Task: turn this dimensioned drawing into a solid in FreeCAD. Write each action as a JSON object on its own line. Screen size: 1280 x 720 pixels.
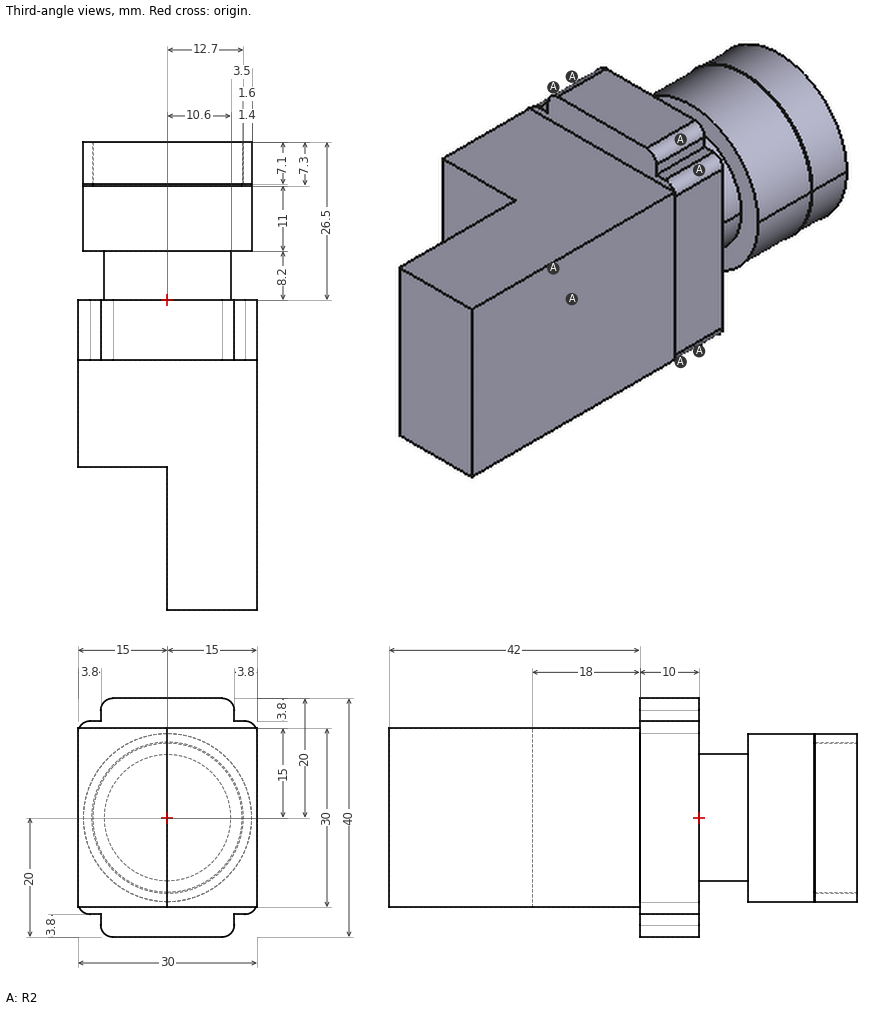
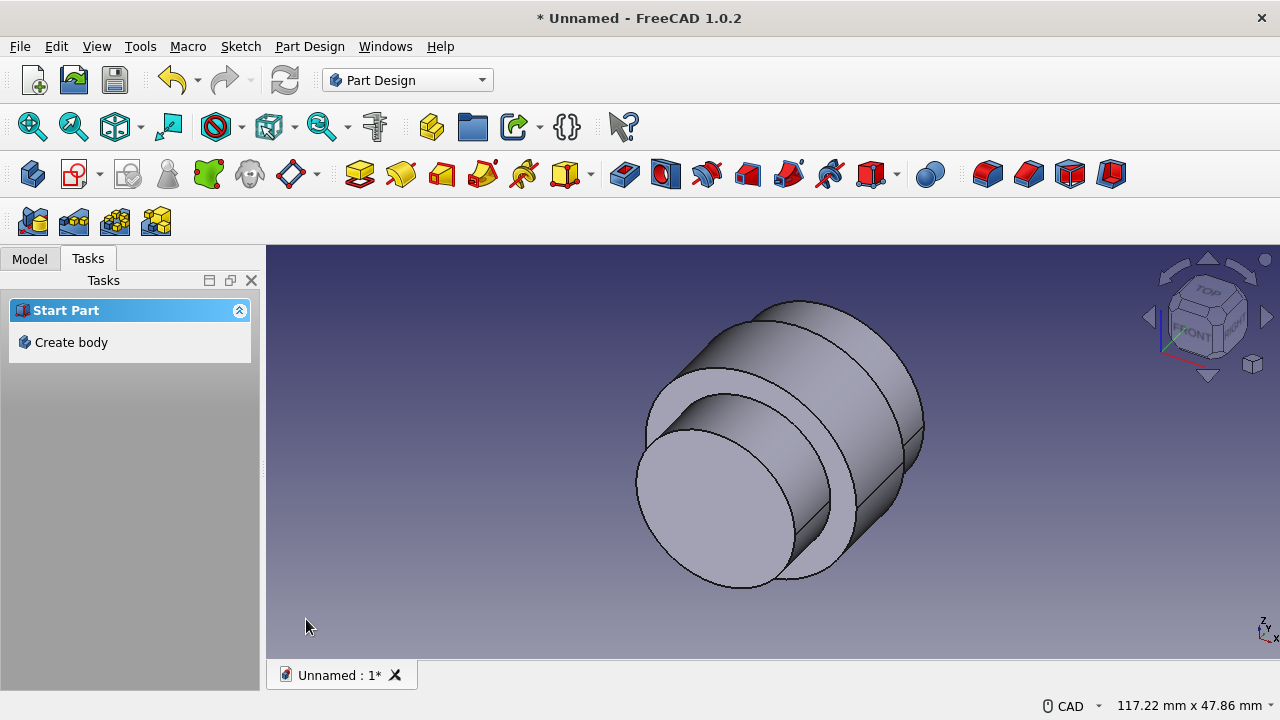
{"action": "left_click", "coordinate": [74, 174]}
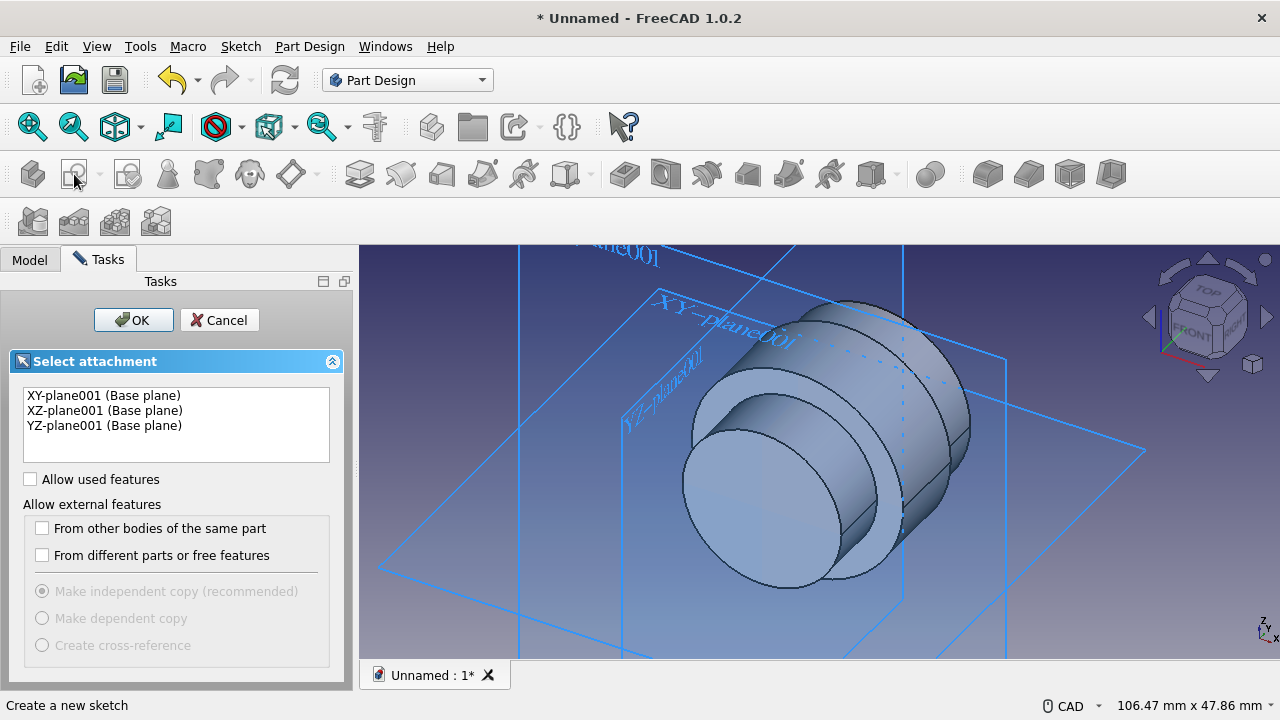
{"action": "left_click", "coordinate": [84, 410]}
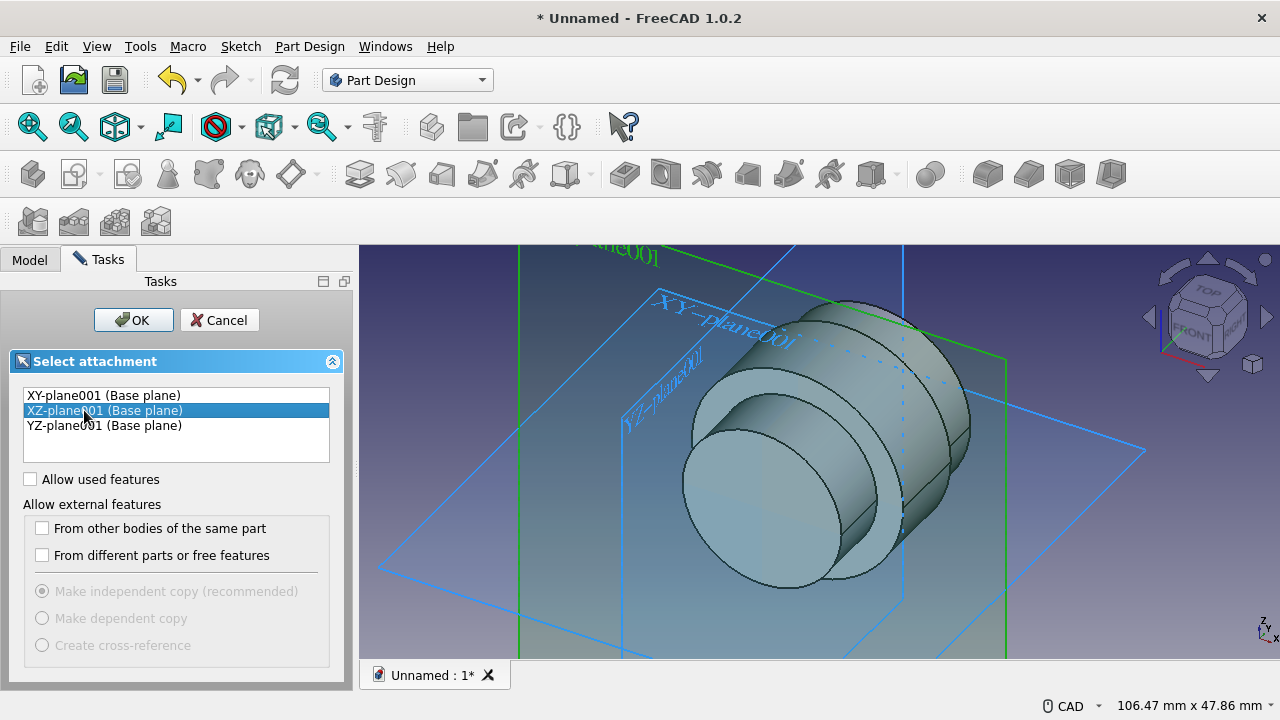
{"action": "left_click", "coordinate": [134, 320]}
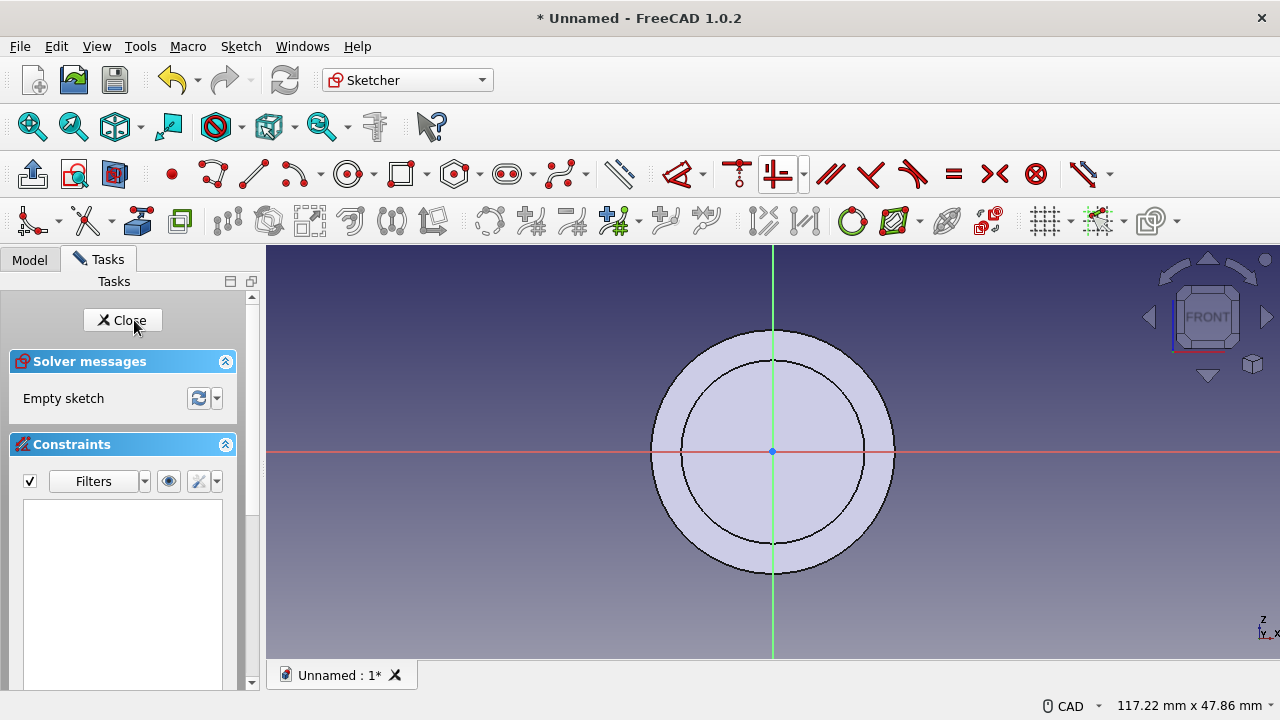
{"action": "scroll", "coordinate": [565, 452], "scroll_direction": "down", "scroll_amount": 2}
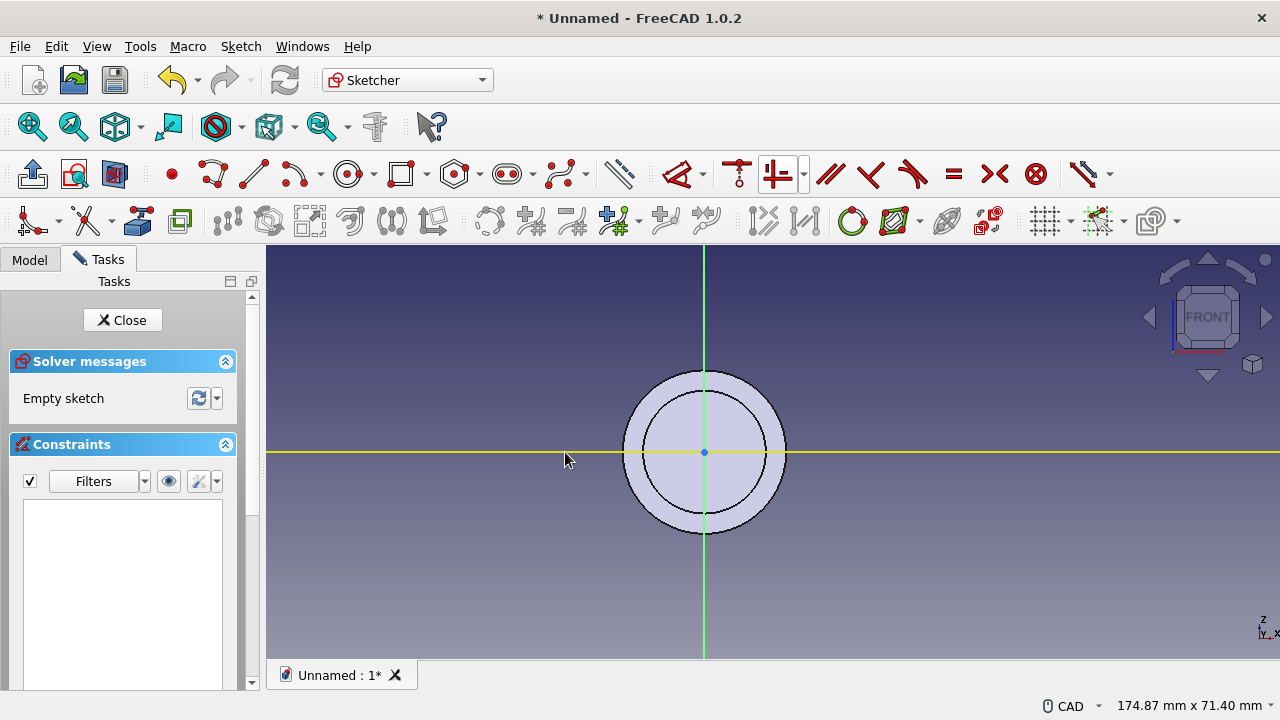
{"action": "key", "text": "g v"}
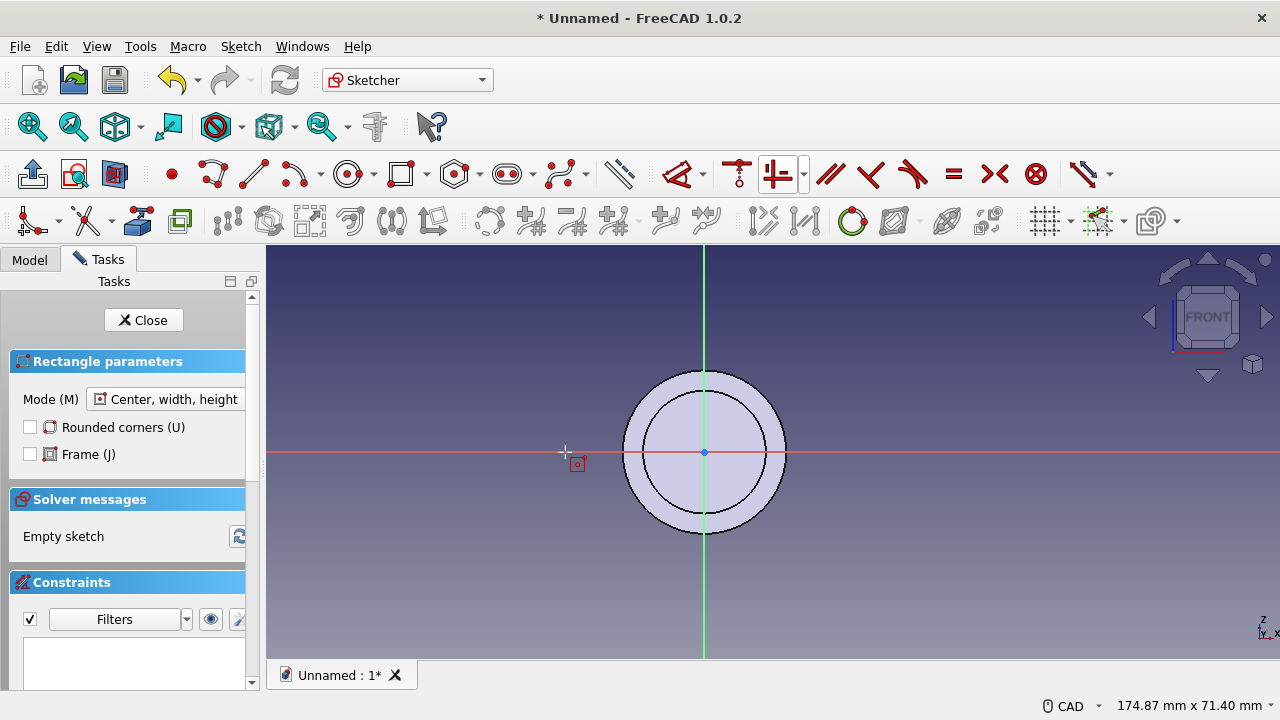
{"action": "left_click", "coordinate": [704, 452]}
{"action": "mouse_move", "coordinate": [791, 336]}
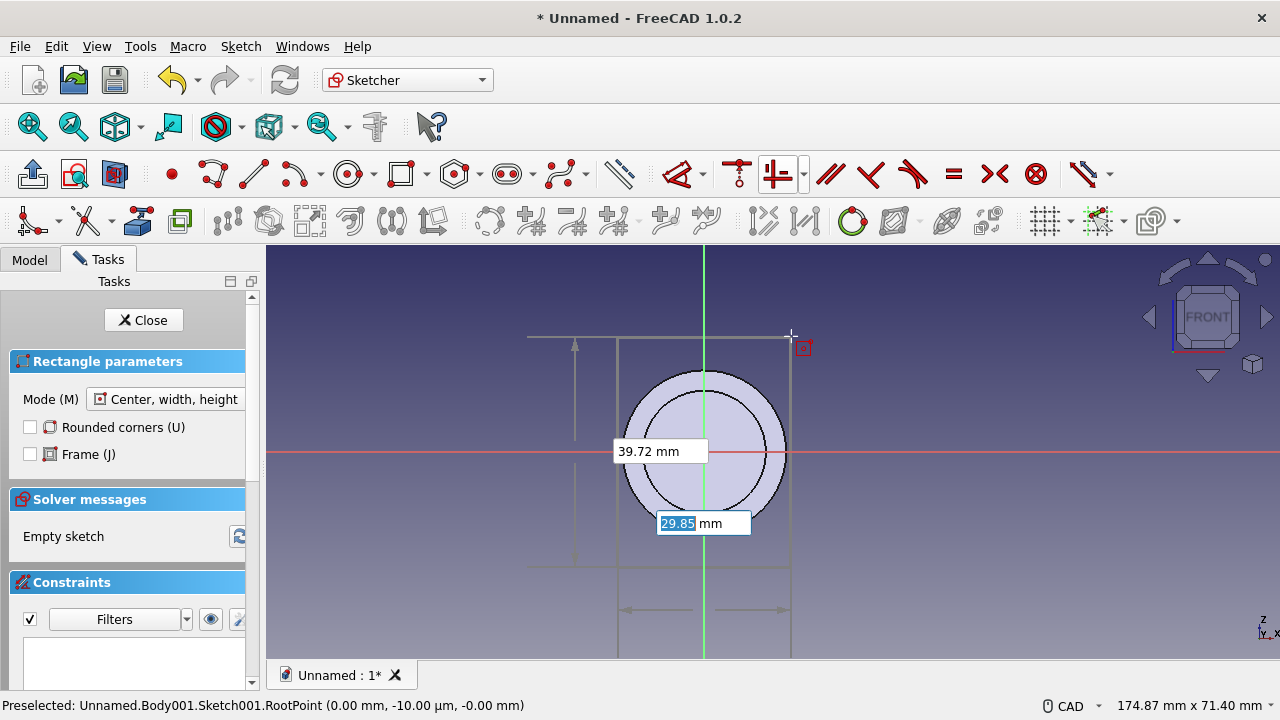
{"action": "type", "text": "30"}
{"action": "key", "text": "Tab"}
{"action": "type", "text": "40"}
{"action": "key", "text": "Return"}
{"action": "key", "text": "Escape"}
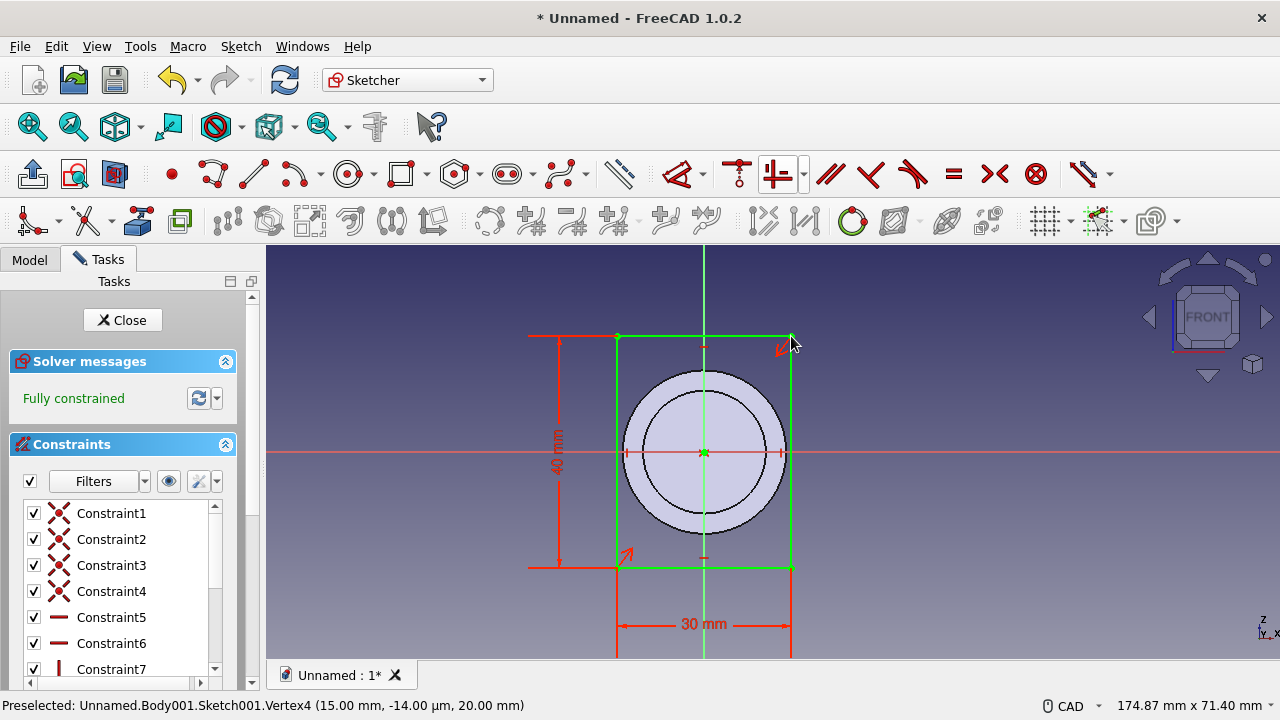
{"action": "left_click", "coordinate": [123, 320]}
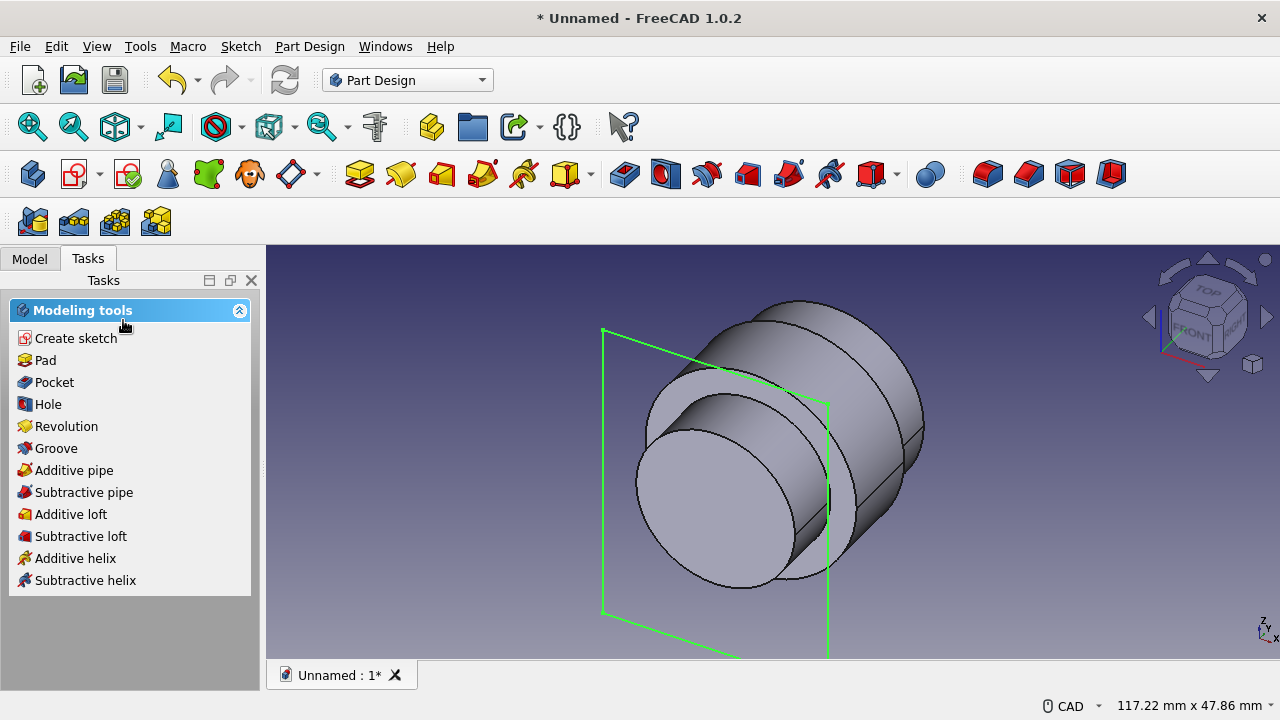
{"action": "left_click", "coordinate": [360, 174]}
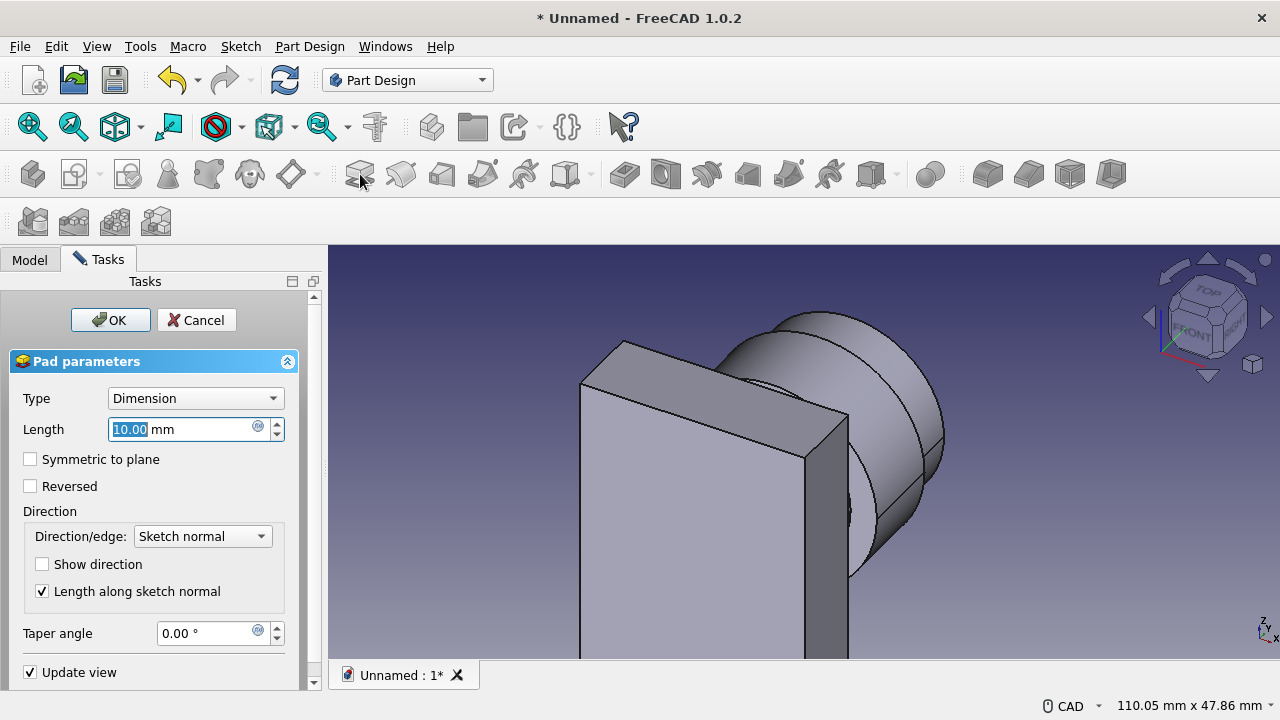
{"action": "type", "text": "10"}
{"action": "key", "text": "Tab"}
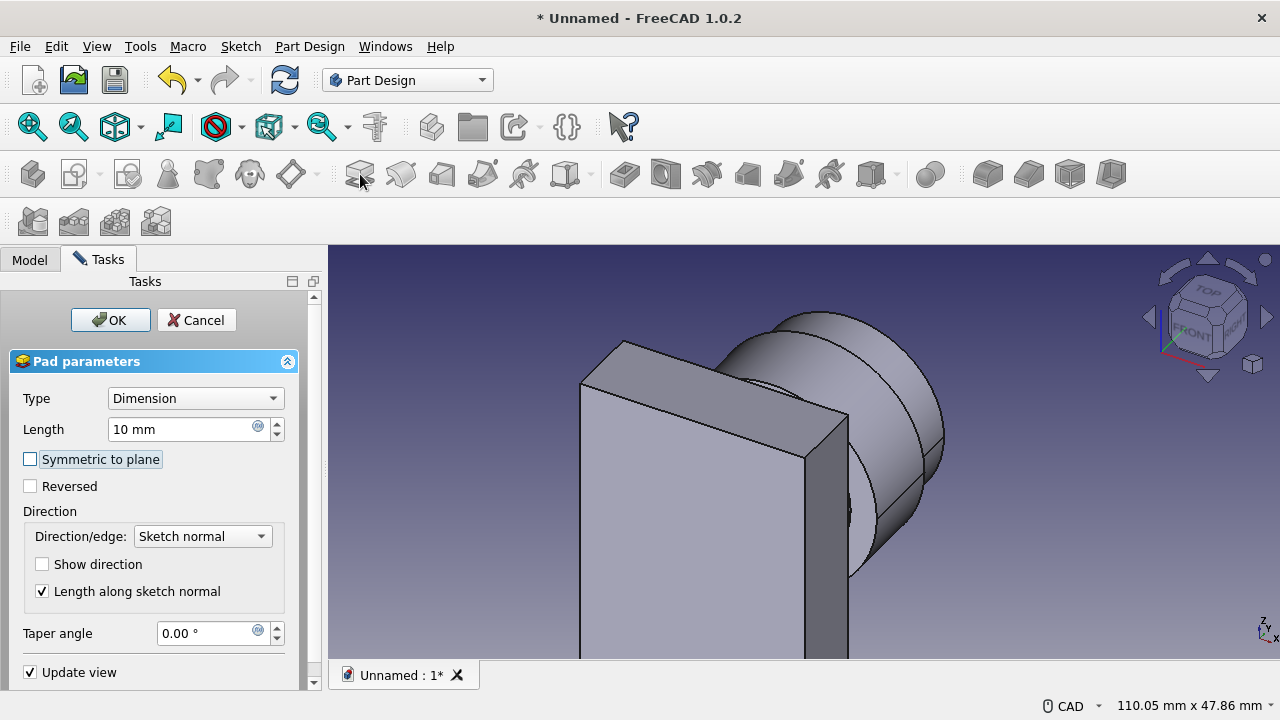
{"action": "left_click", "coordinate": [111, 320]}